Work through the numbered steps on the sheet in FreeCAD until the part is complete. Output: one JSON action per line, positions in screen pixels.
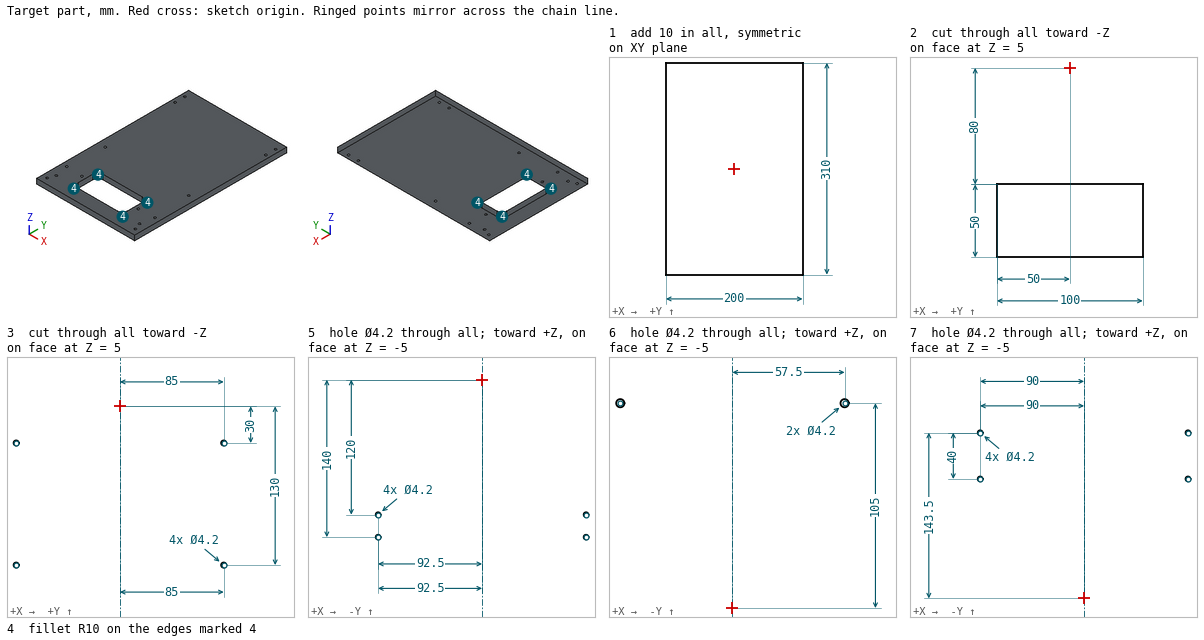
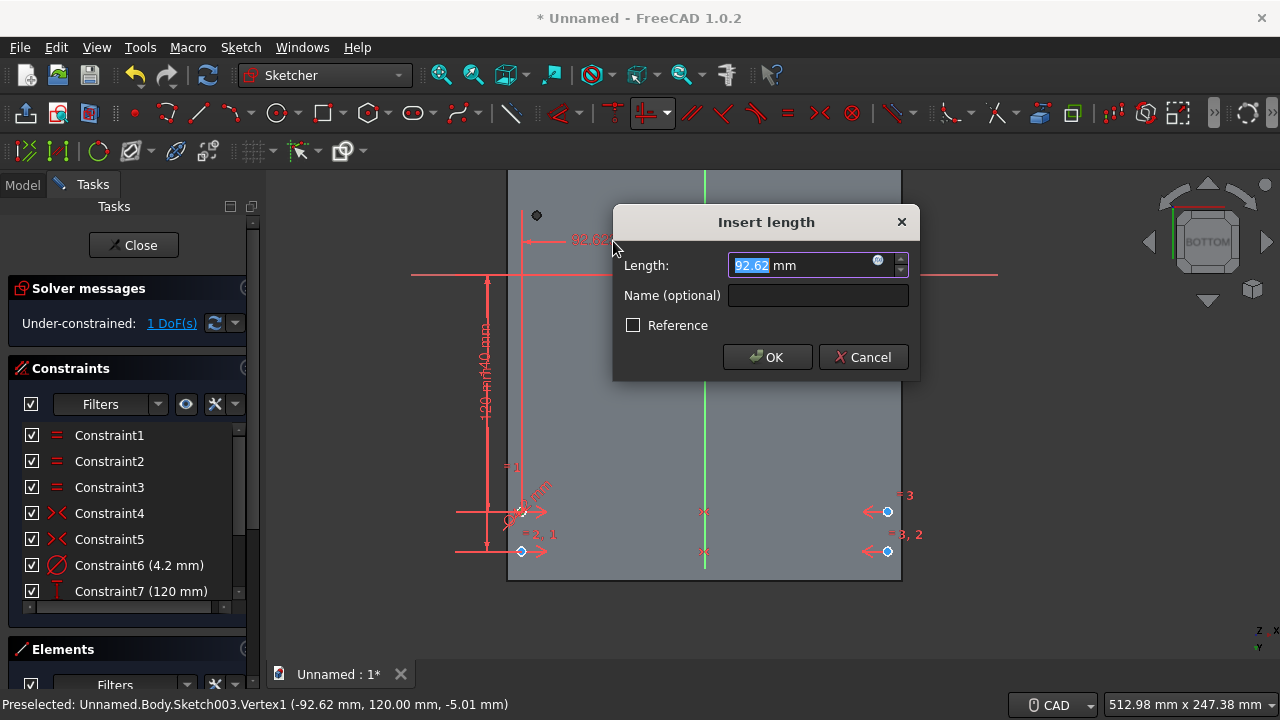
{"action": "type", "text": "92.5"}
{"action": "key", "text": "Return"}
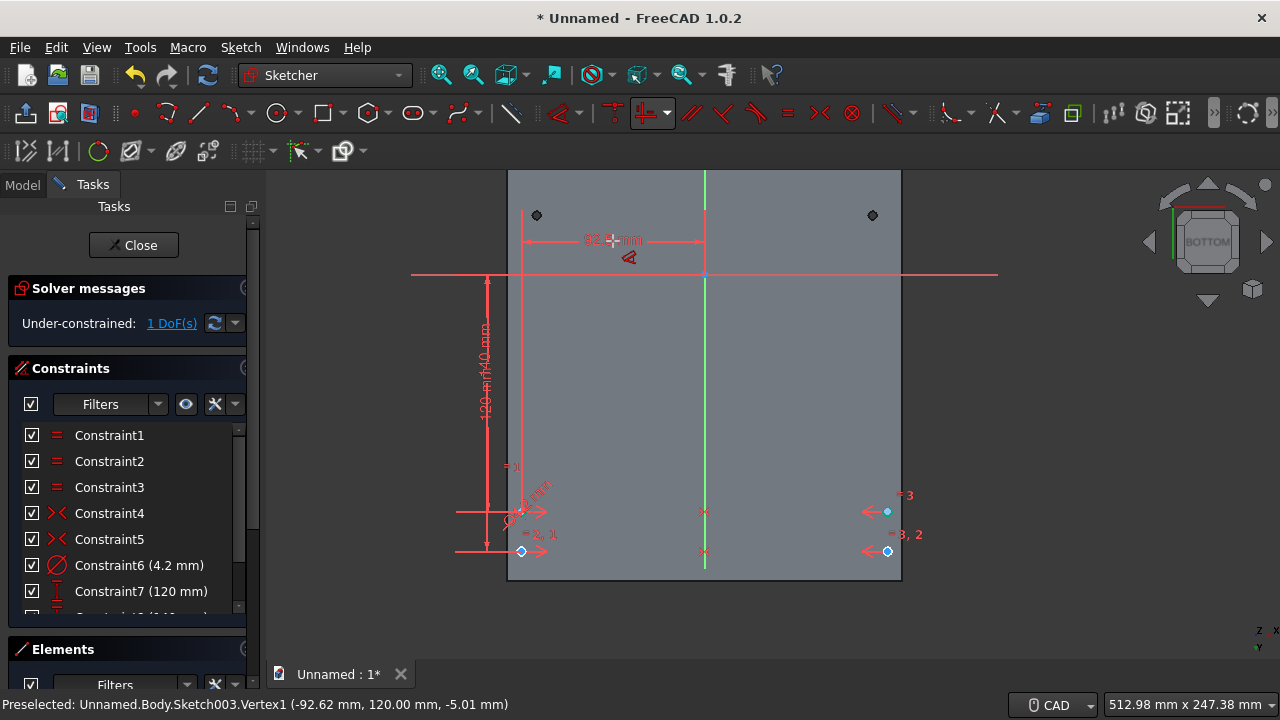
{"action": "left_click", "coordinate": [521, 552]}
{"action": "left_click", "coordinate": [613, 586]}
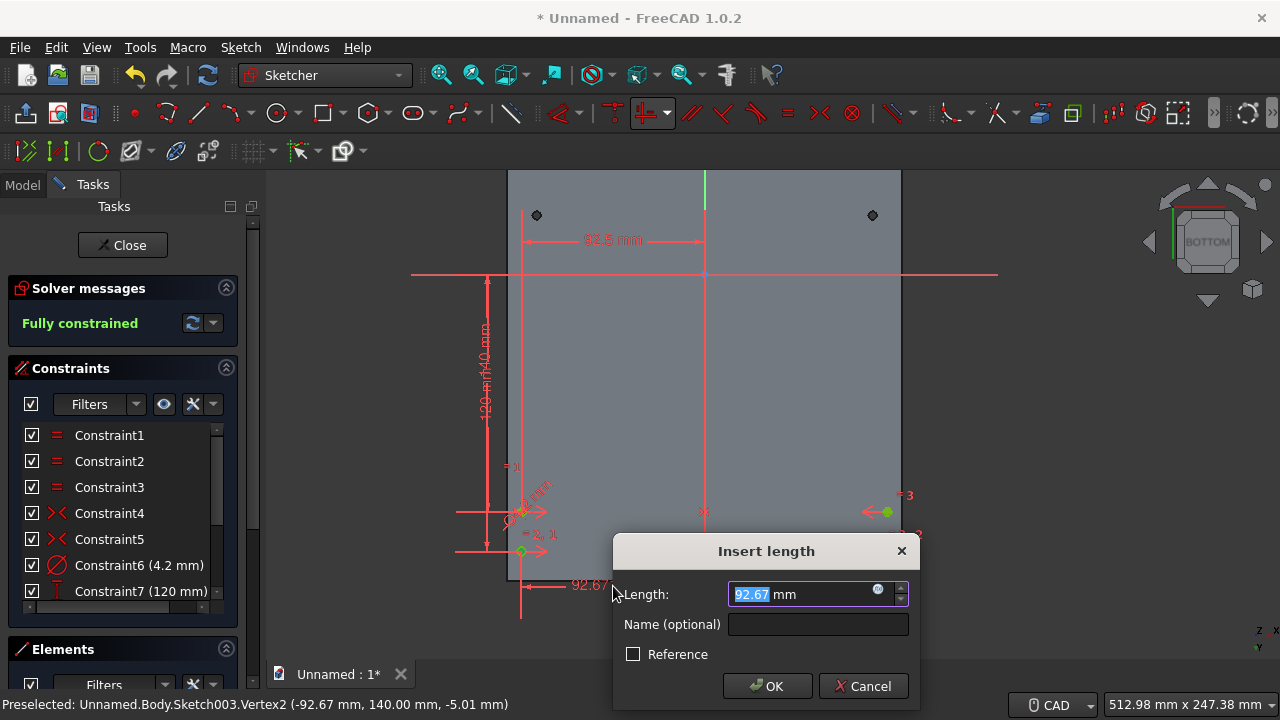
{"action": "type", "text": "92.5"}
{"action": "key", "text": "Return"}
{"action": "key", "text": "Escape"}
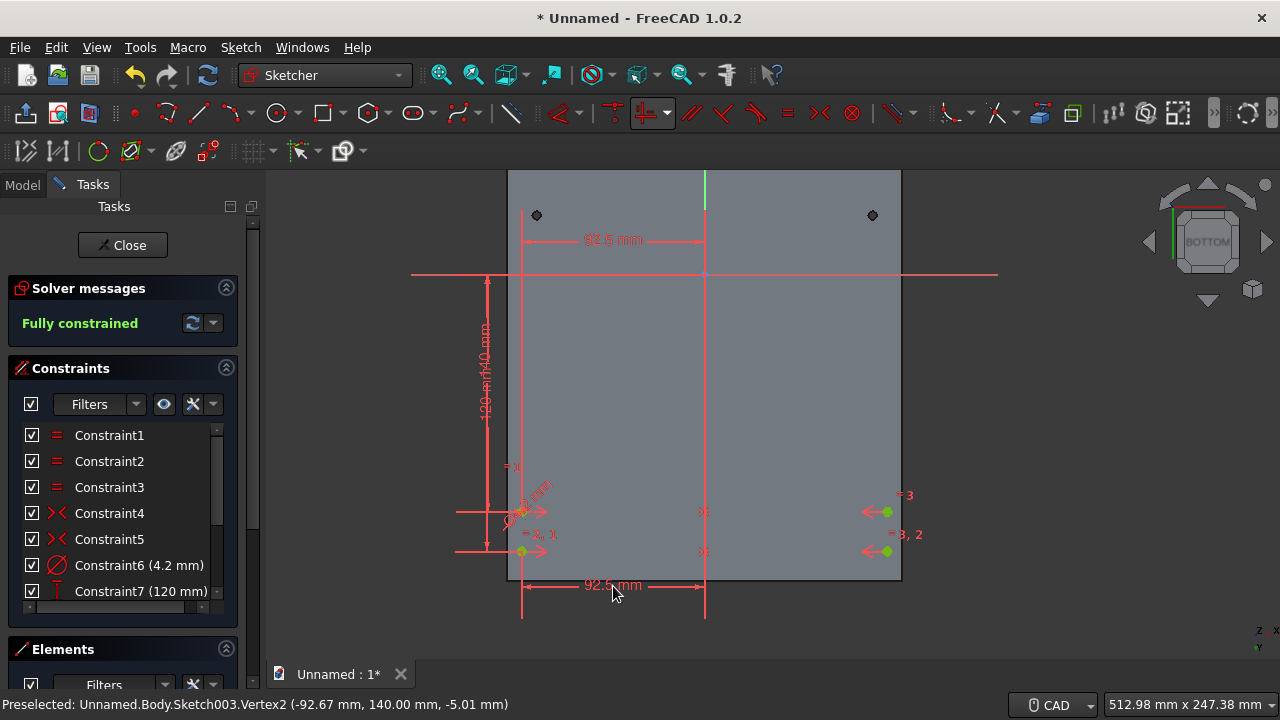
{"action": "left_click", "coordinate": [123, 245]}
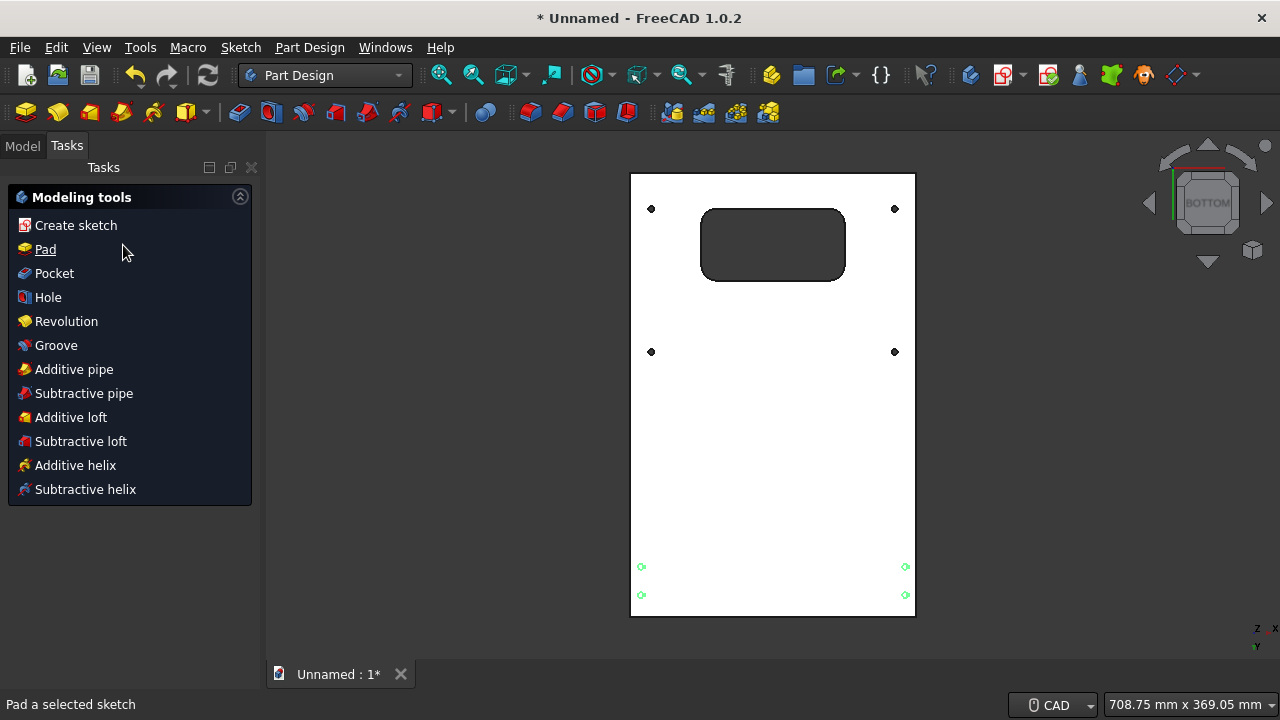
{"action": "left_click", "coordinate": [272, 112]}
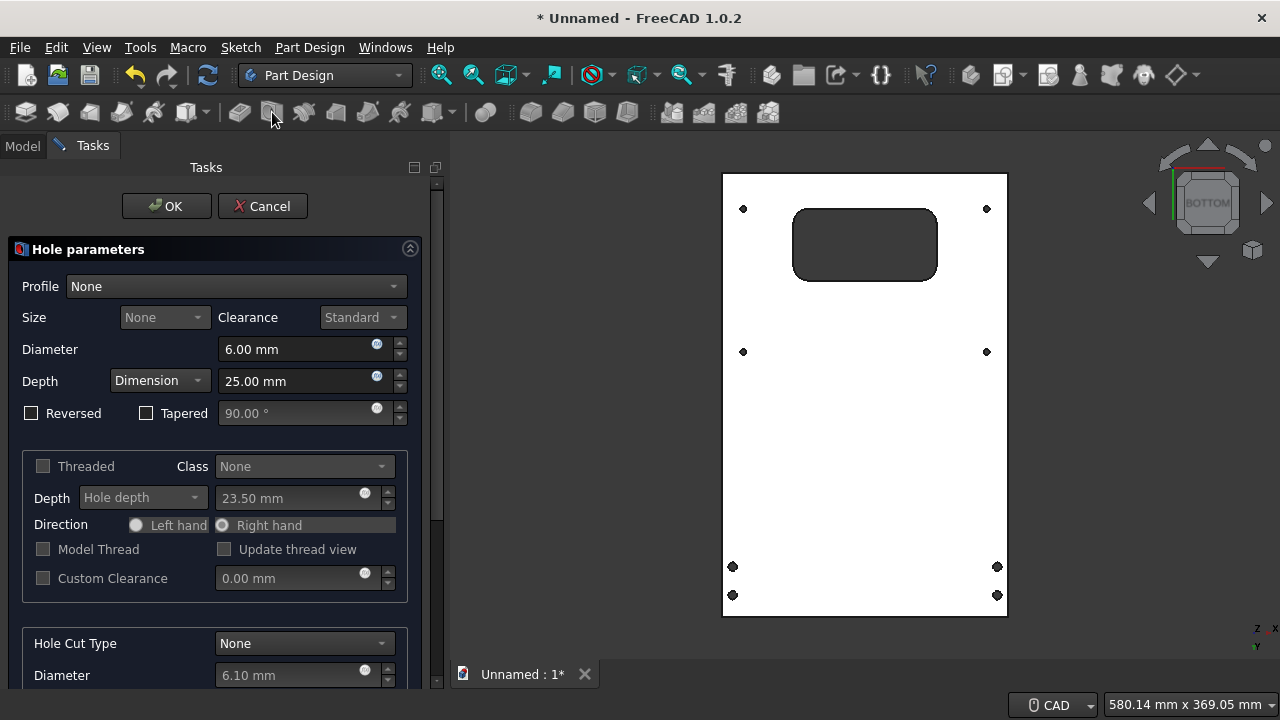
{"action": "triple_click", "coordinate": [305, 349]}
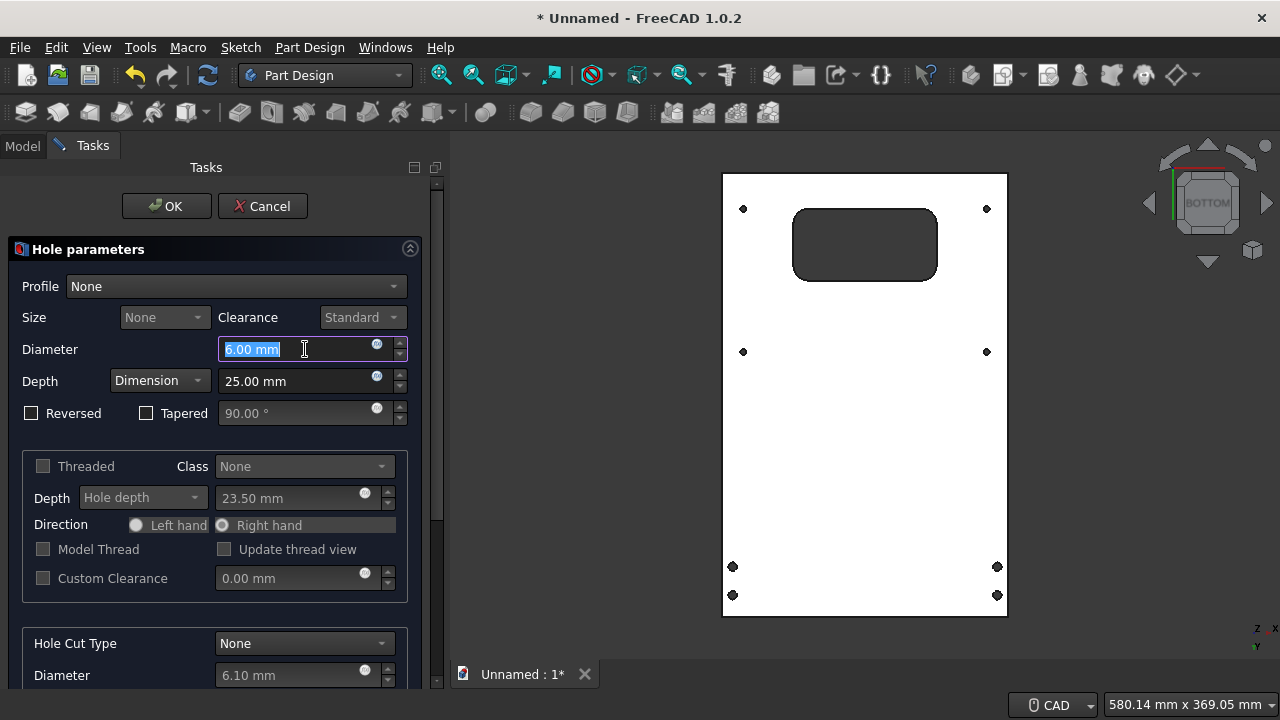
{"action": "type", "text": "4.2"}
{"action": "key", "text": "Tab"}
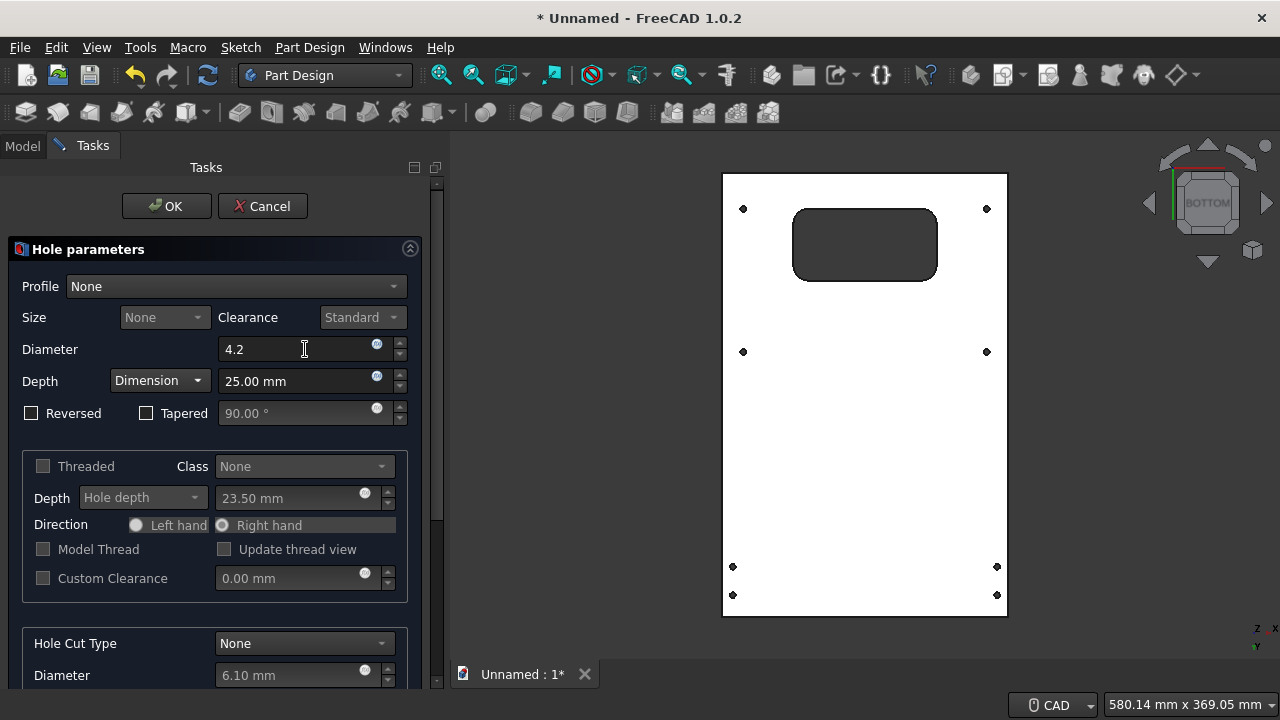
{"action": "left_click", "coordinate": [161, 380]}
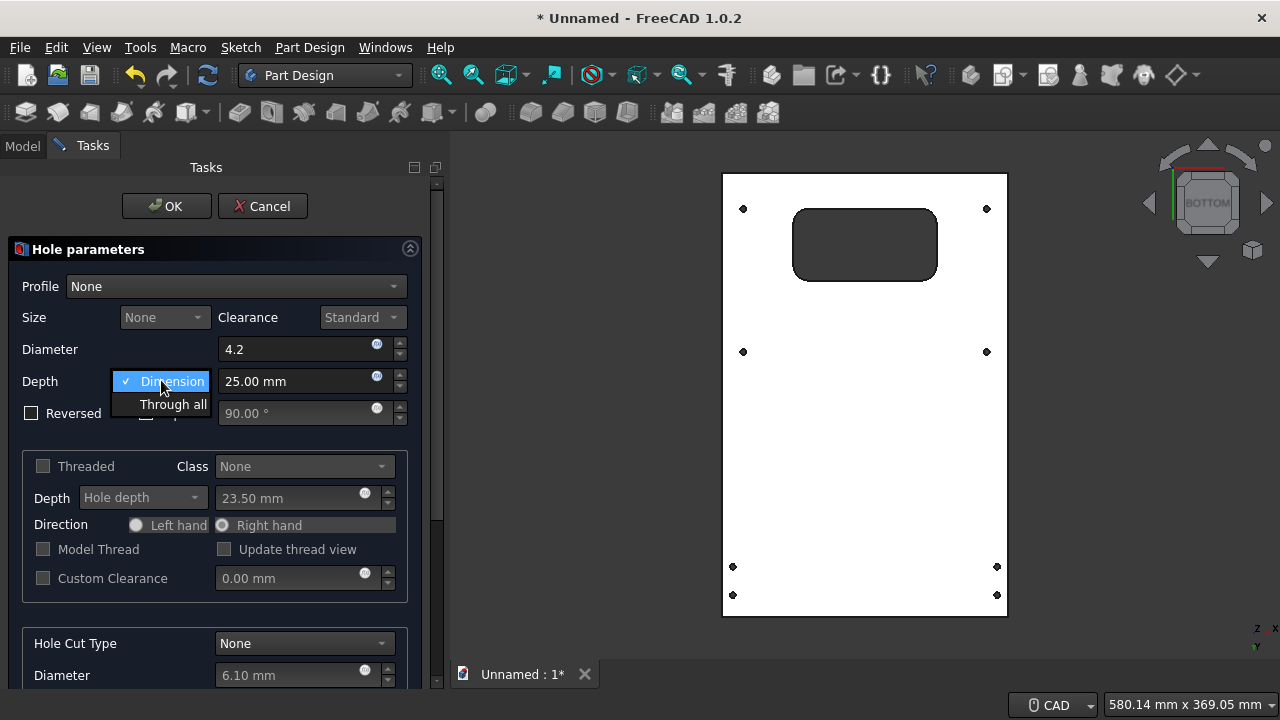
{"action": "left_click", "coordinate": [160, 404]}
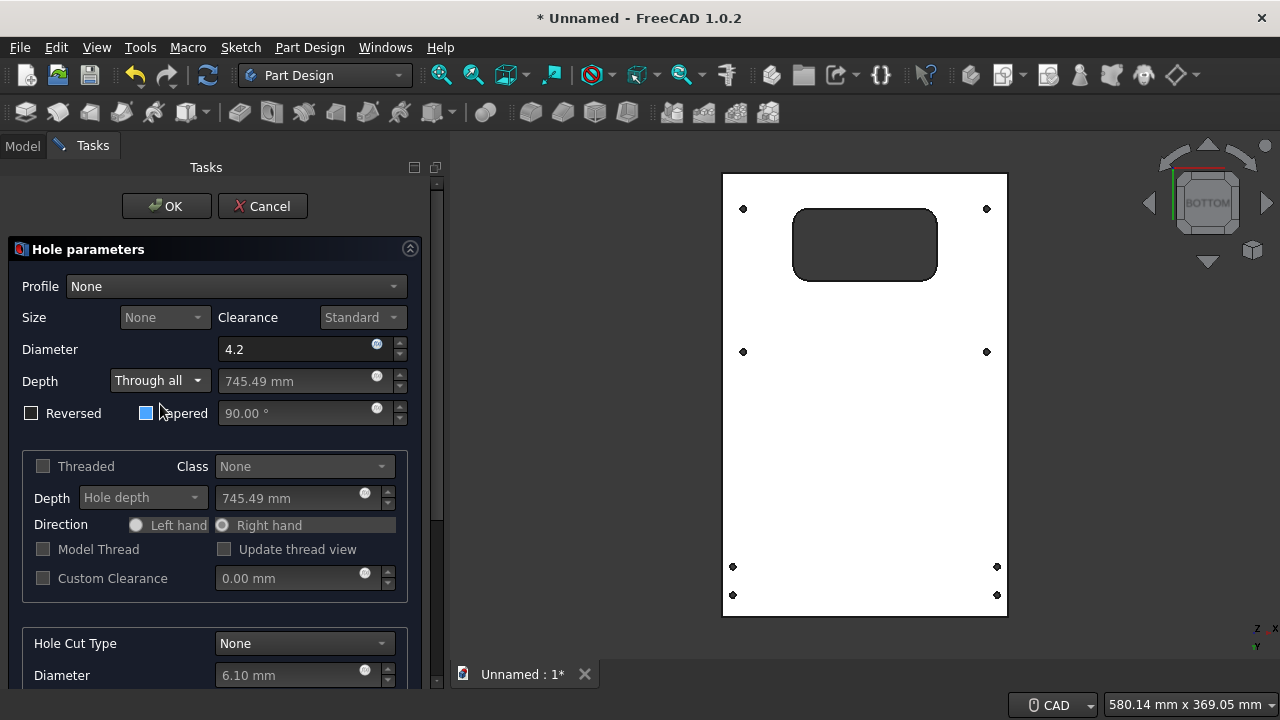
{"action": "left_click", "coordinate": [167, 206]}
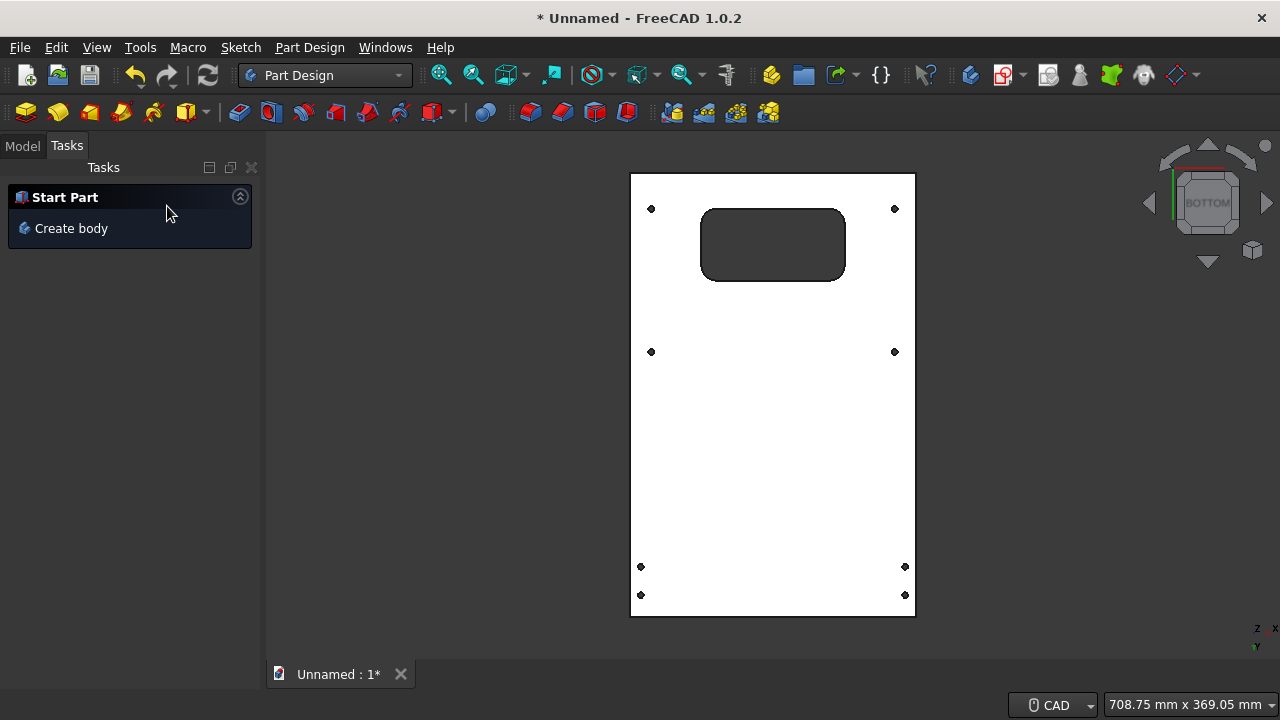
{"action": "left_click", "coordinate": [773, 457]}